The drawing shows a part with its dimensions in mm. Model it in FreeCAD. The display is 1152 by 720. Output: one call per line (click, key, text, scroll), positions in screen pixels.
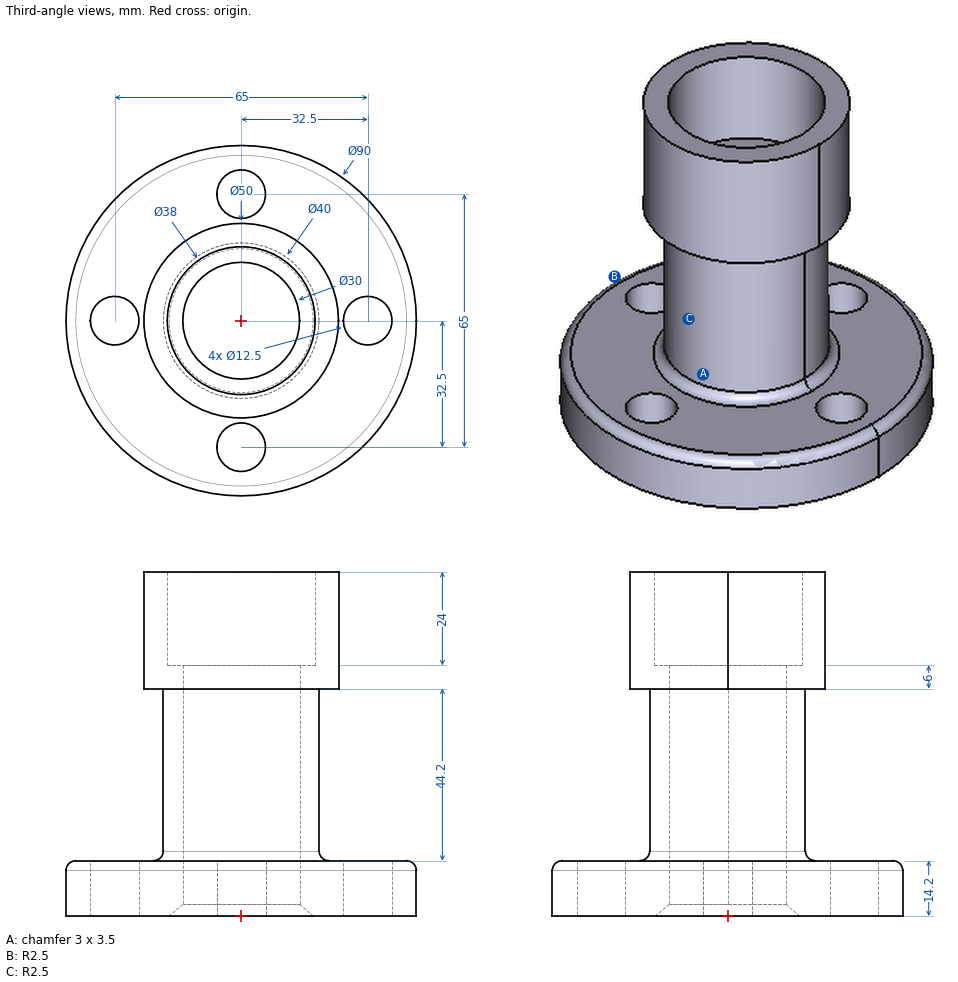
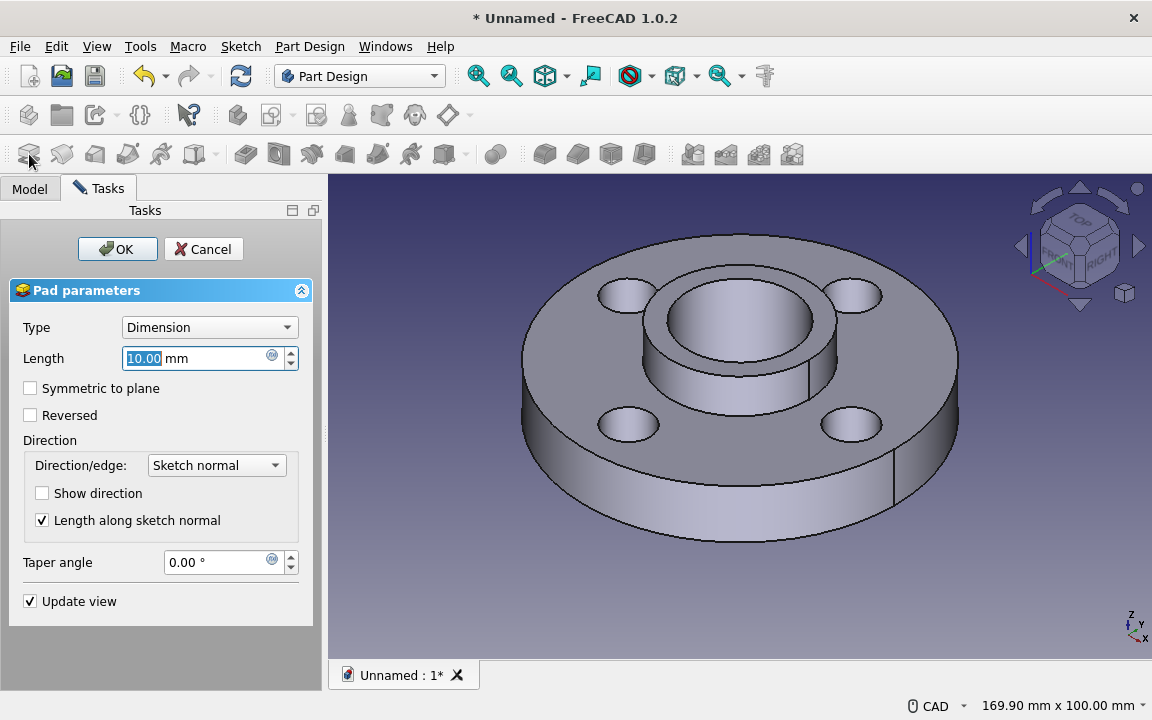
text(44.2)
key(Tab)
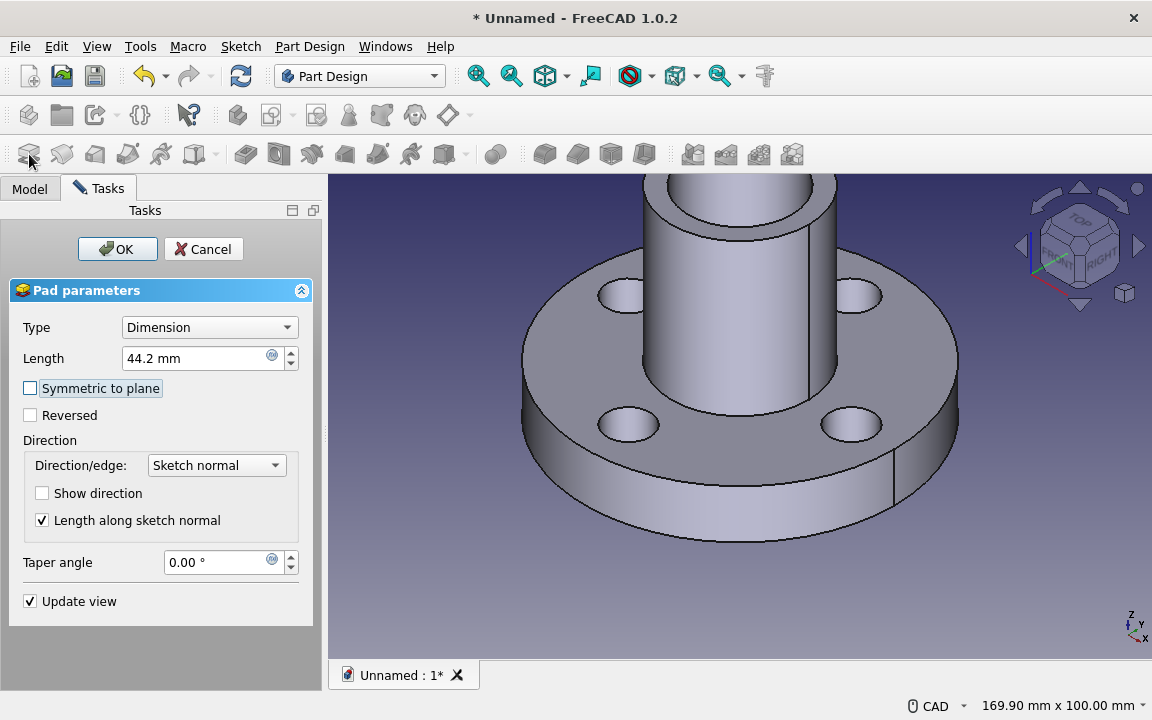
click(118, 249)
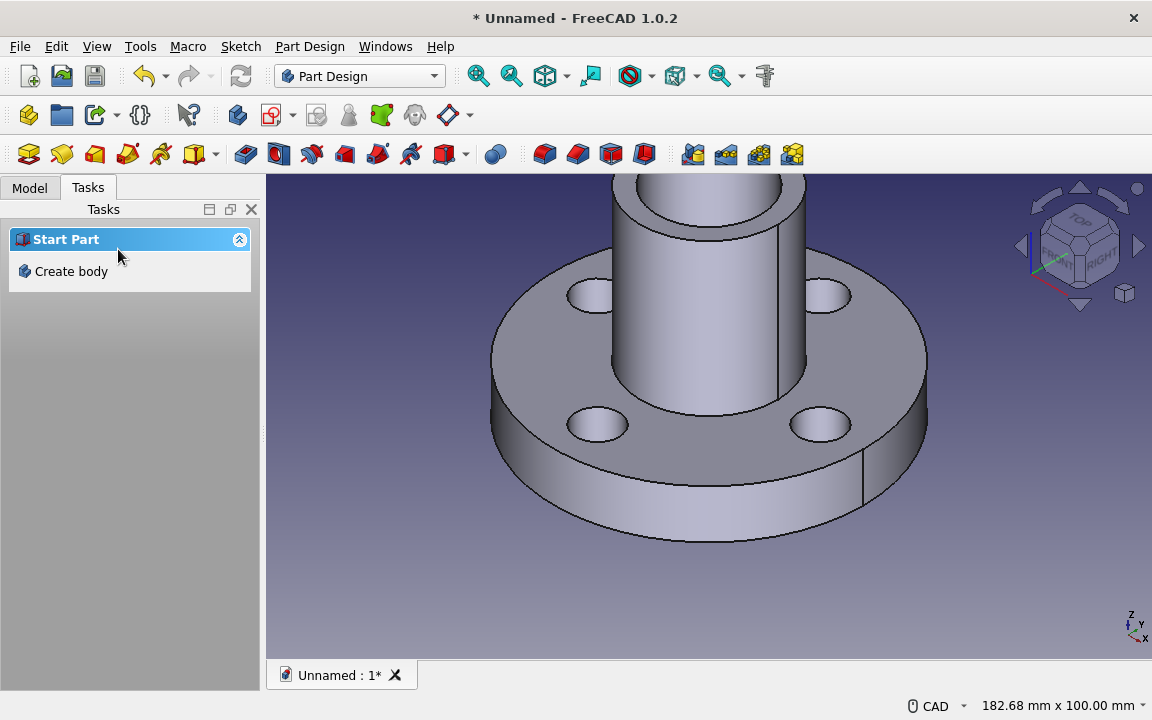
click(479, 76)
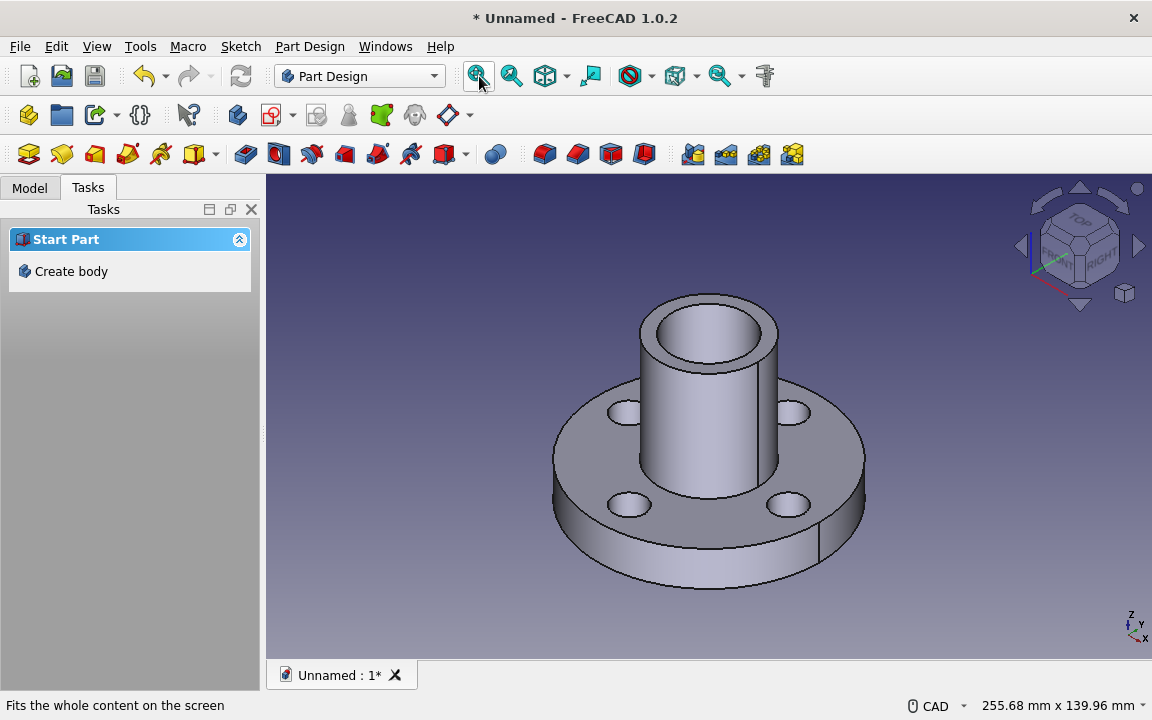
click(570, 499)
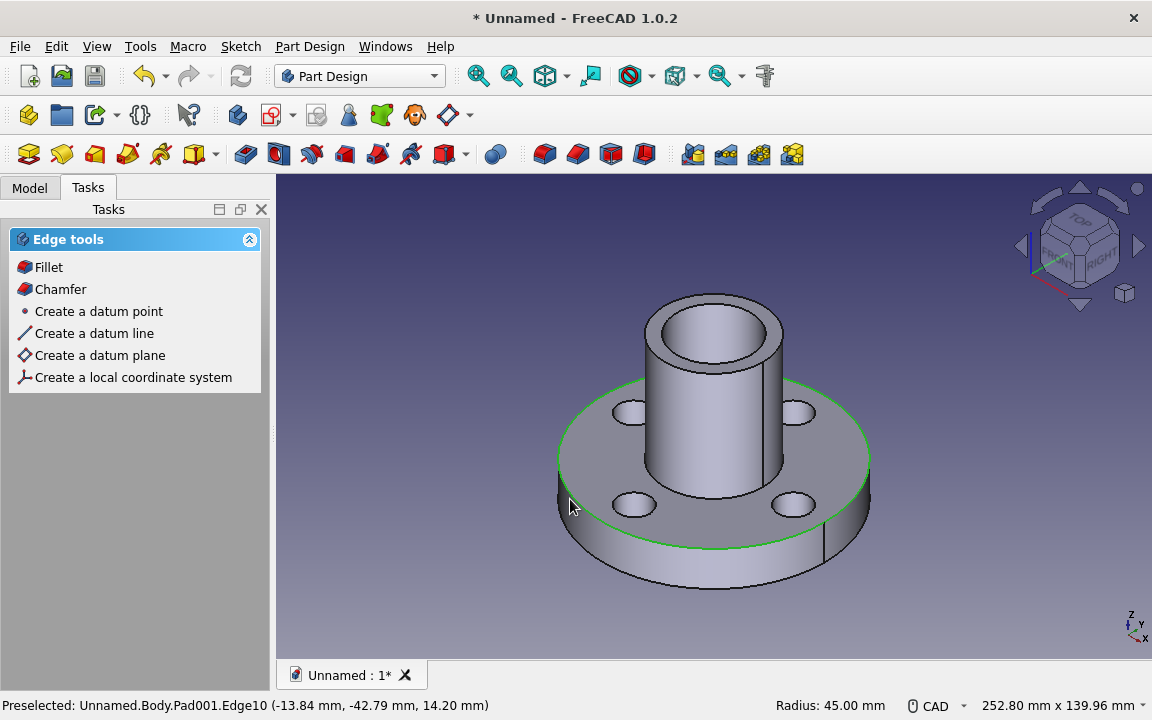
click(545, 154)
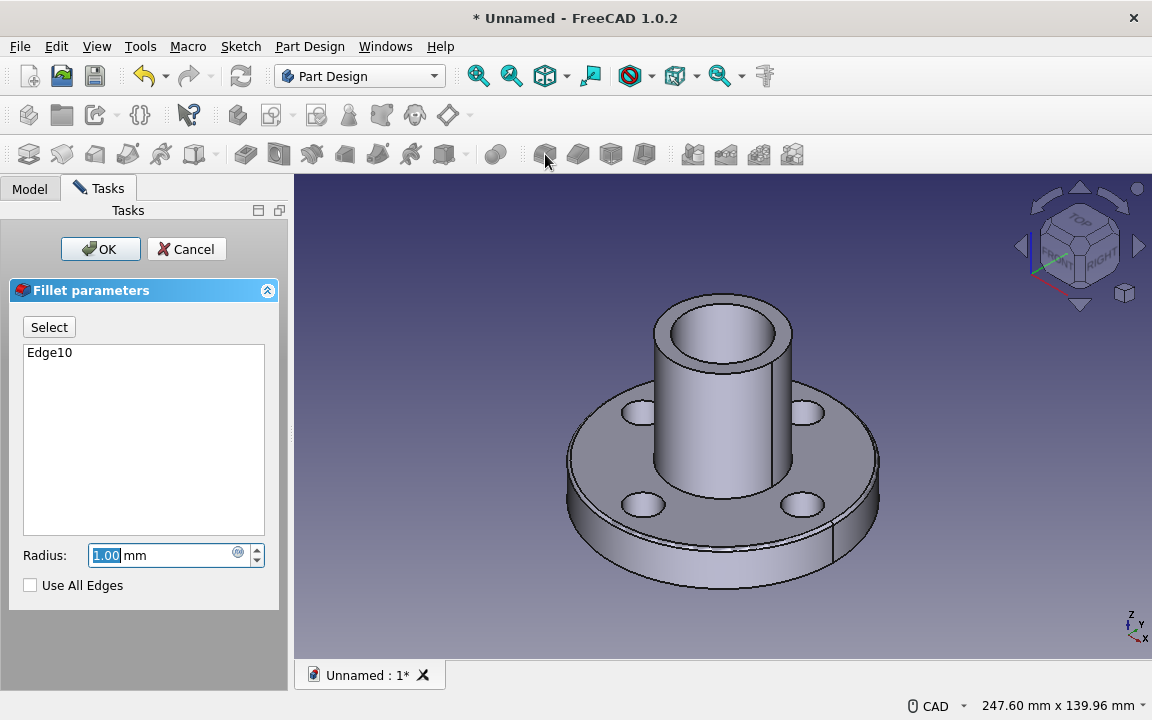
text(2.5)
key(Tab)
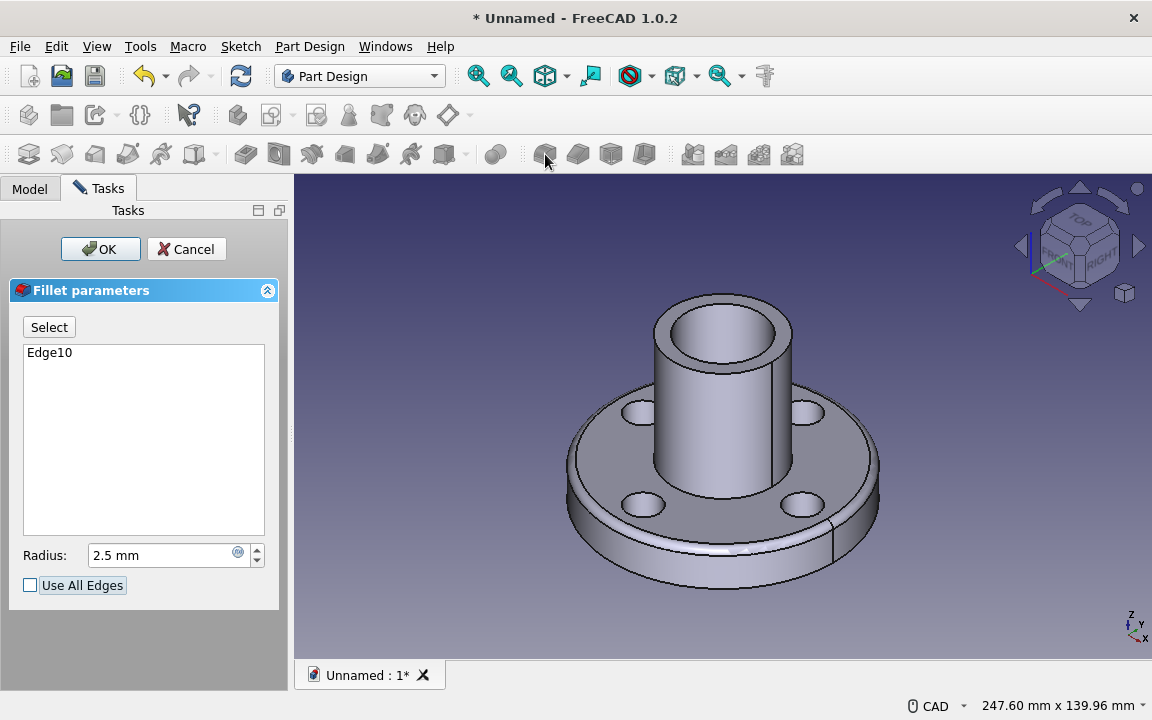
click(101, 249)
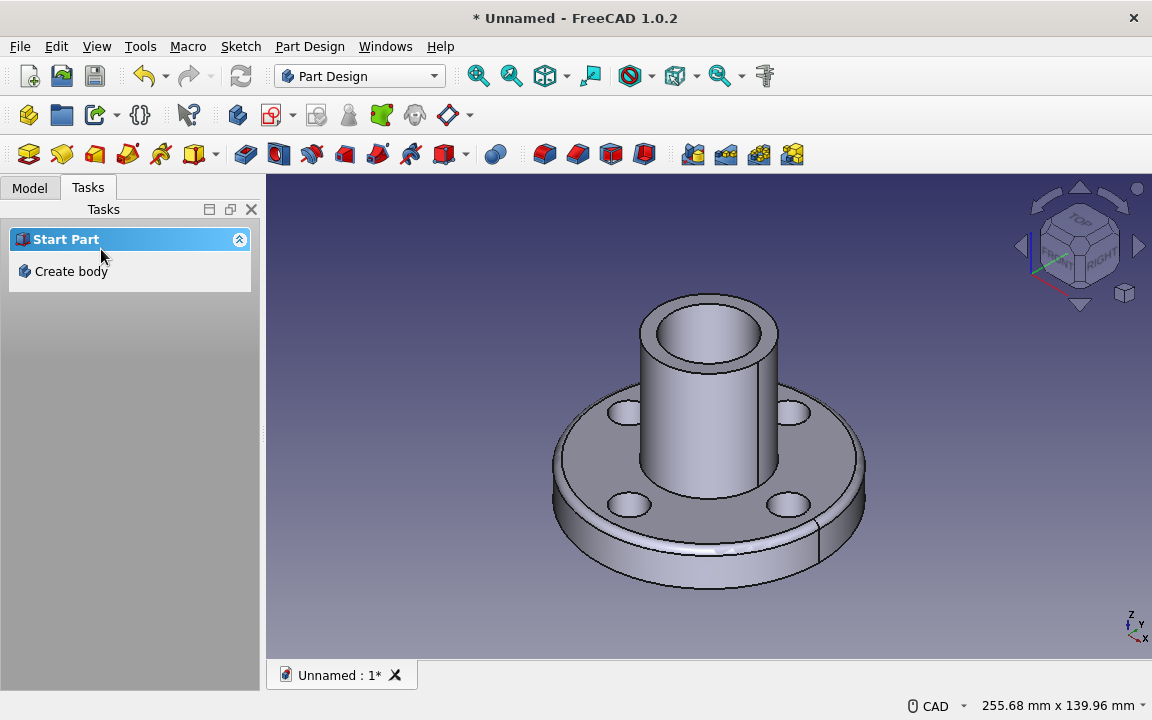
click(653, 317)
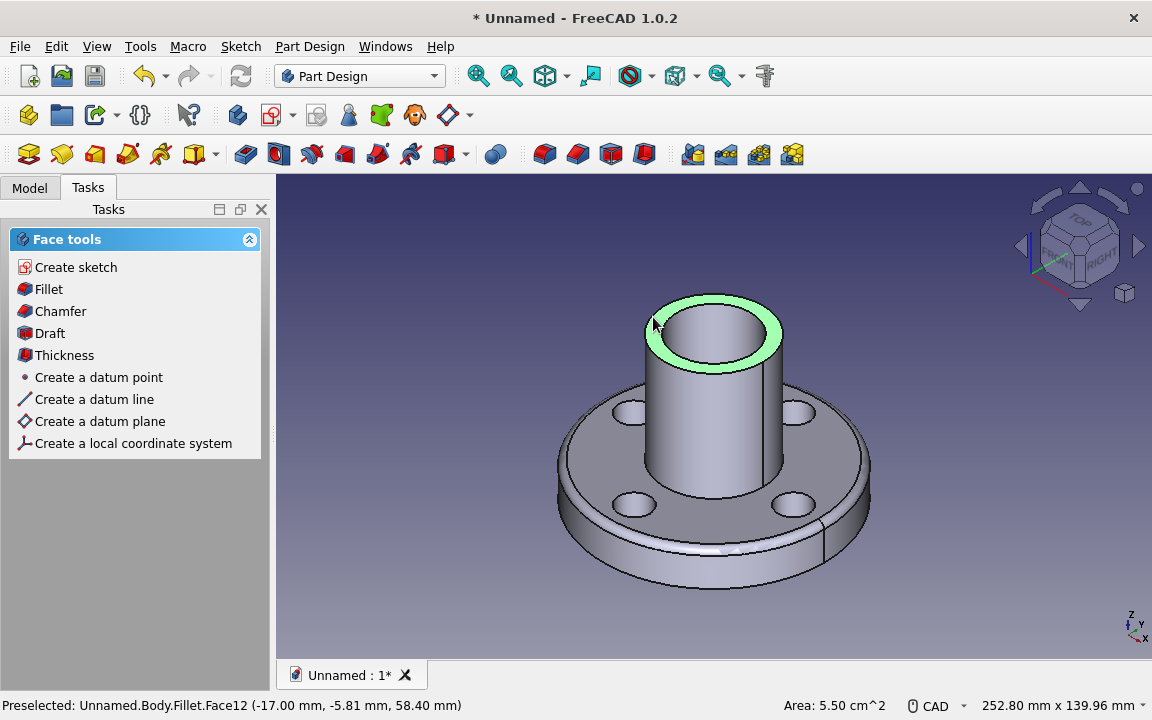
click(270, 116)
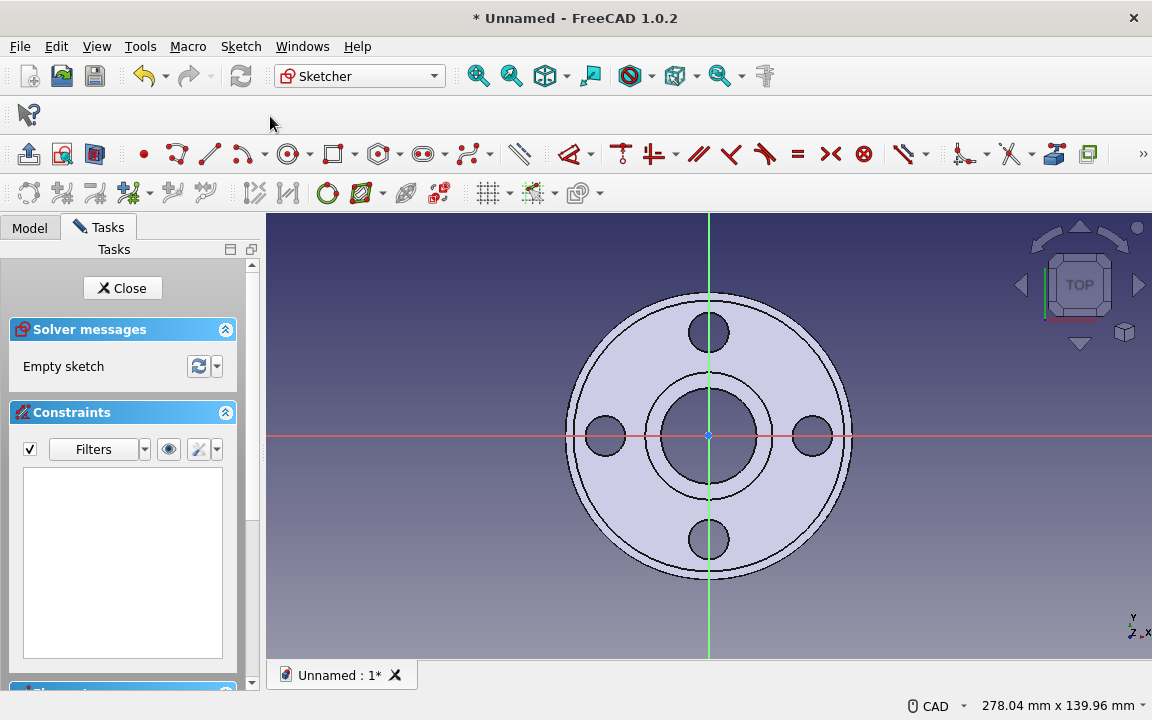
scroll(792, 436, up, 3)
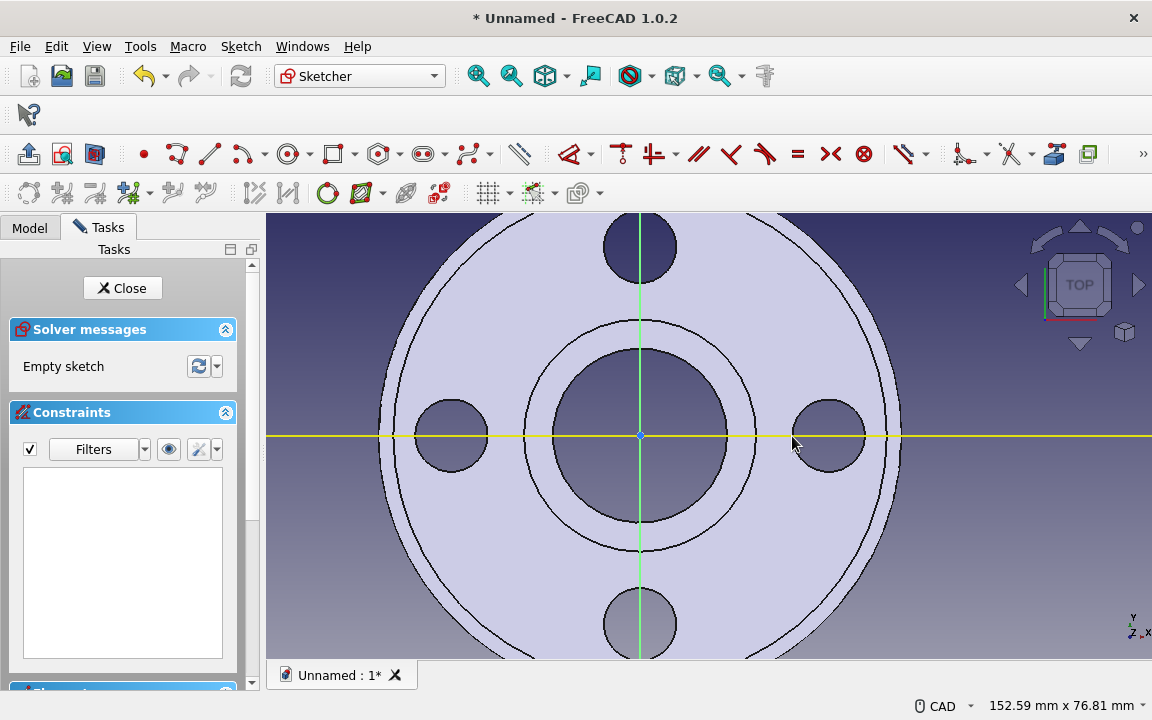
click(288, 154)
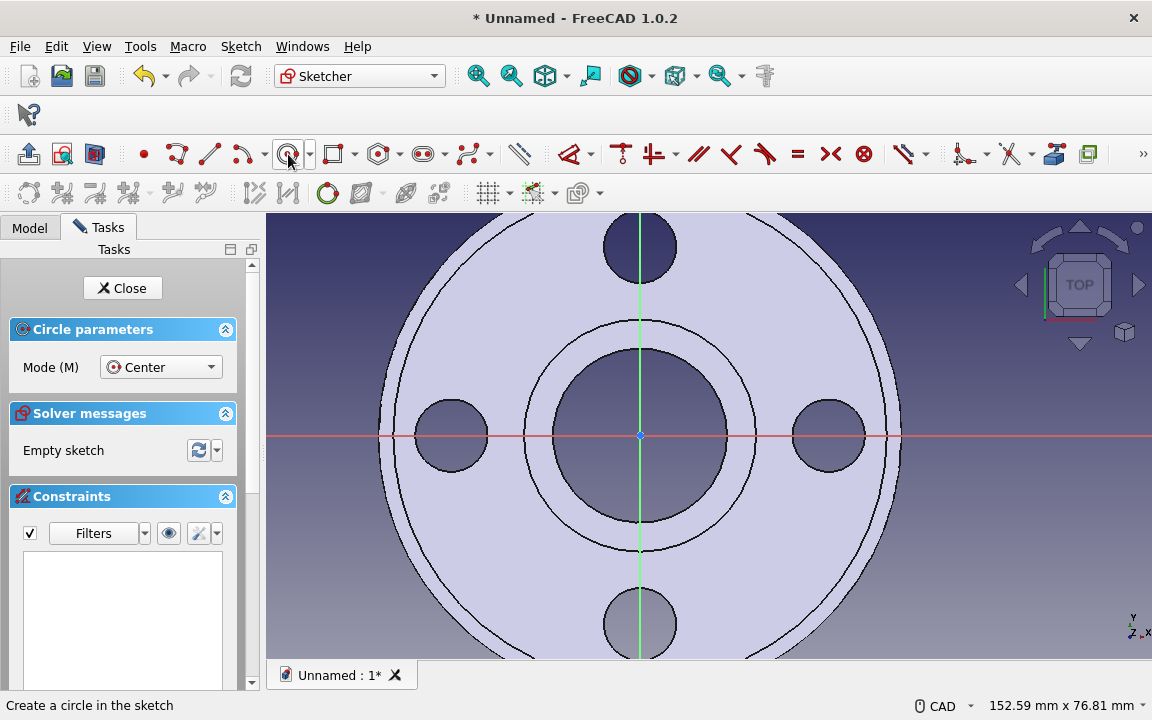
click(640, 436)
click(743, 333)